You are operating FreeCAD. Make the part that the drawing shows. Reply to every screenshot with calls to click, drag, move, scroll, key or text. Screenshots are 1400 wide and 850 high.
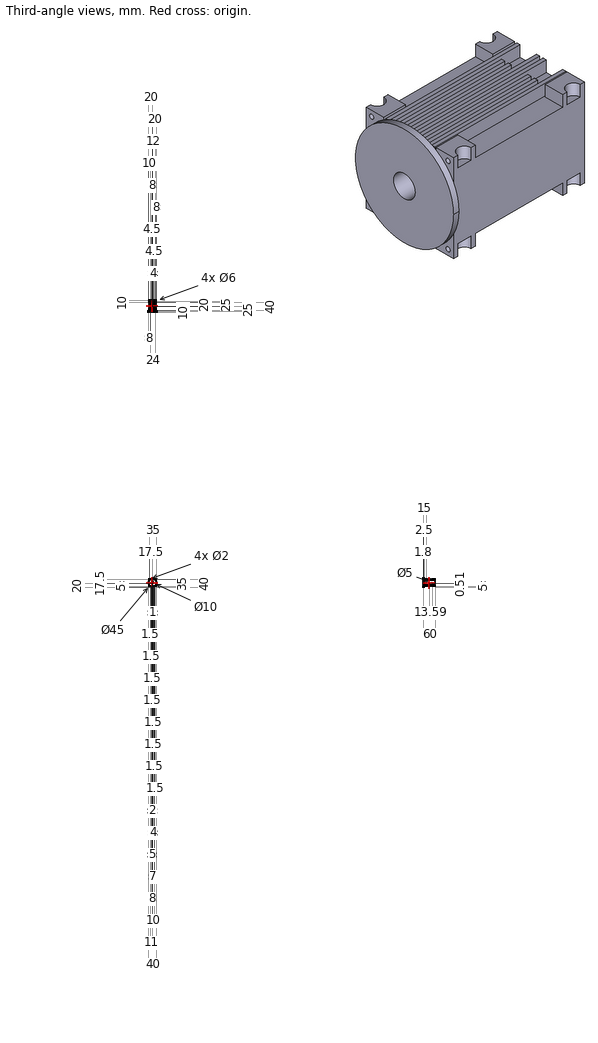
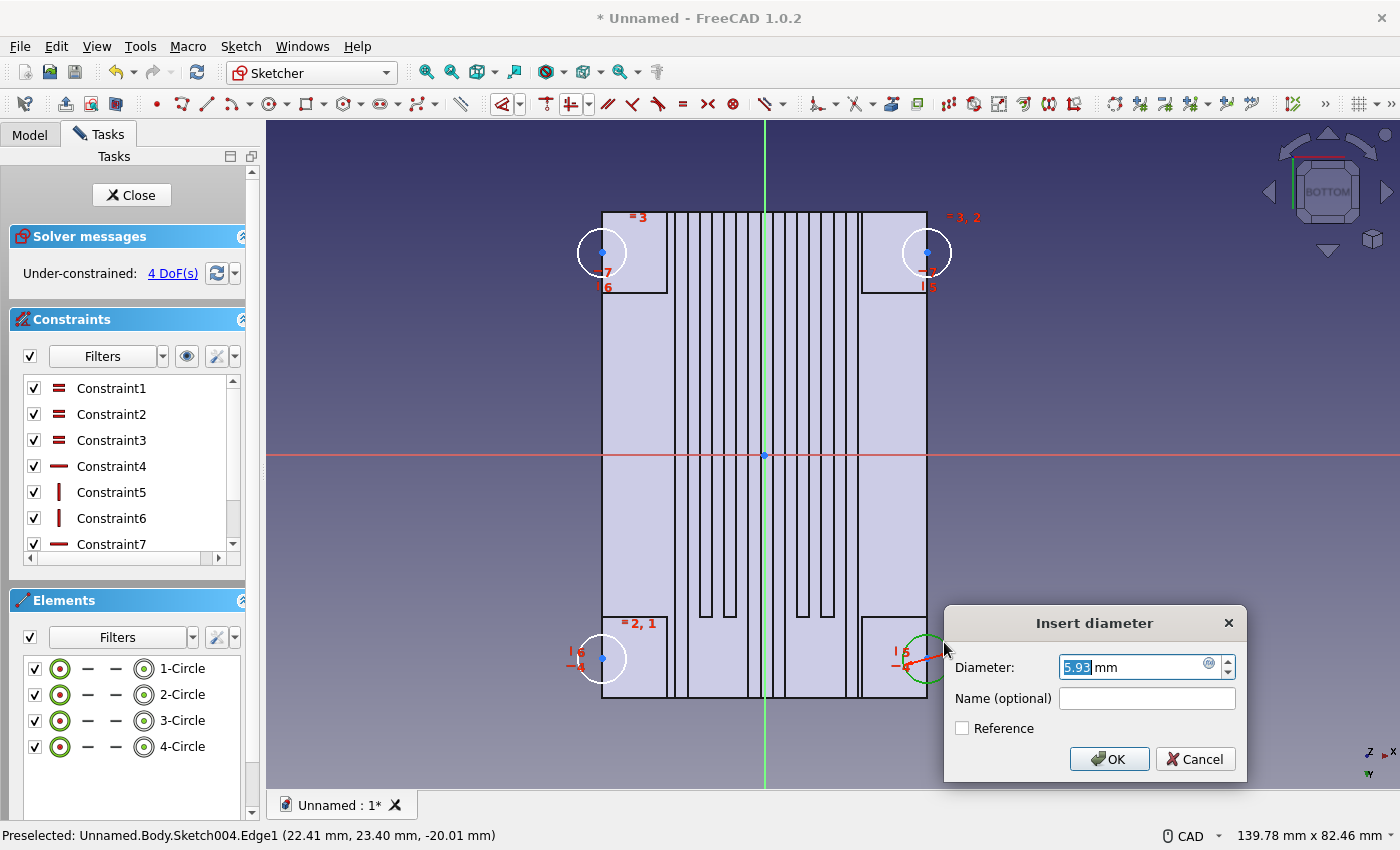
text(6)
key(Return)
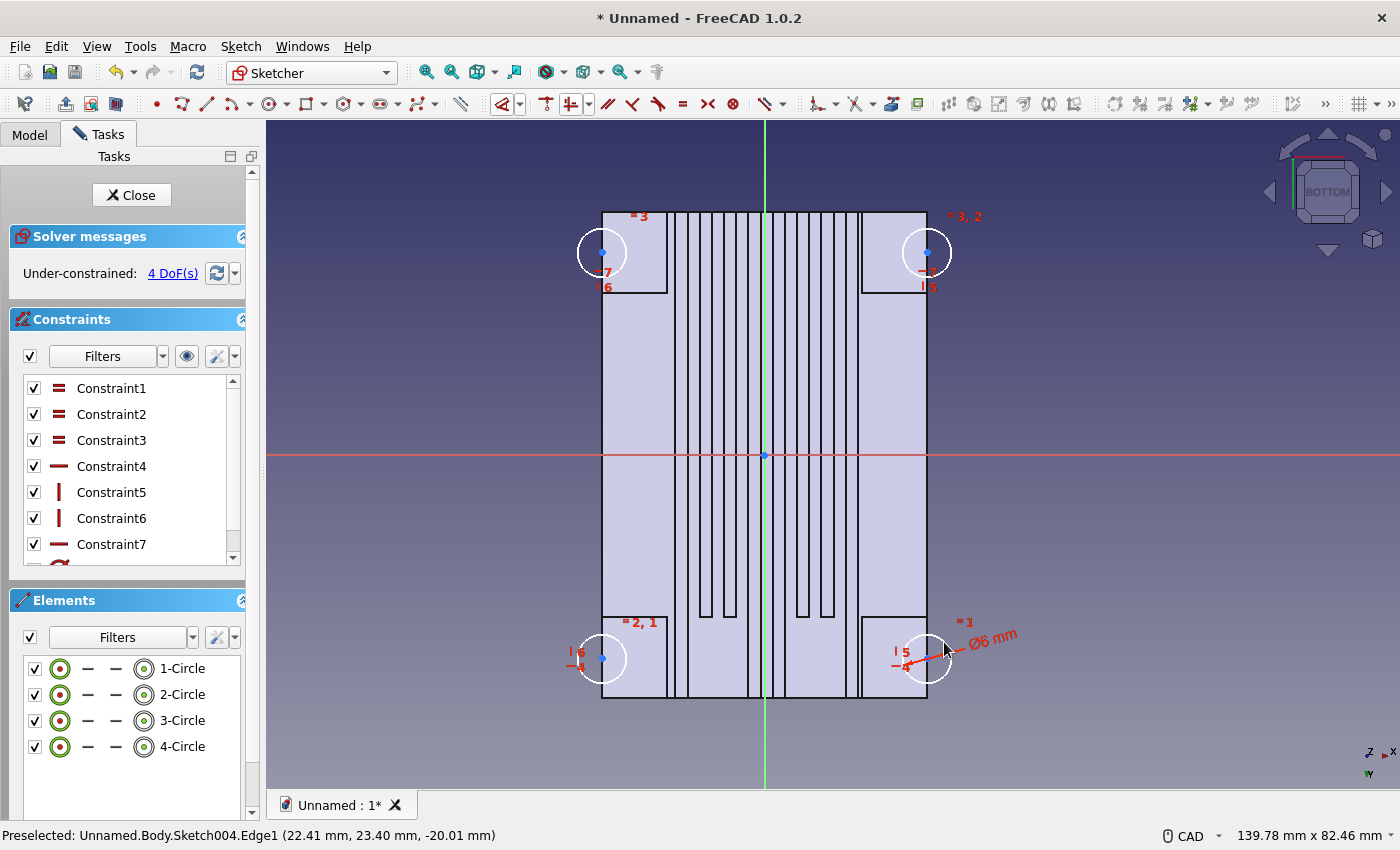
click(927, 659)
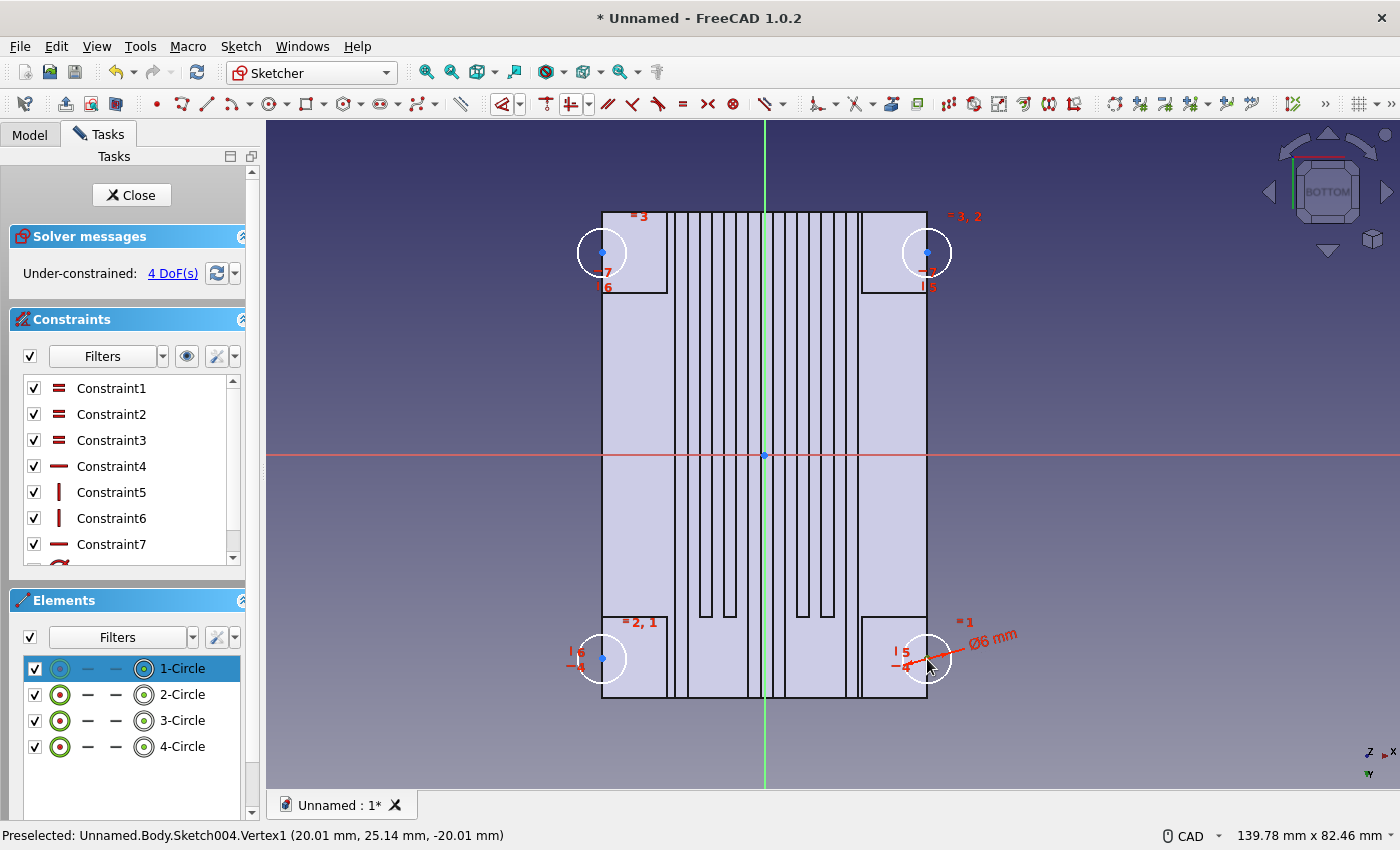
key(l)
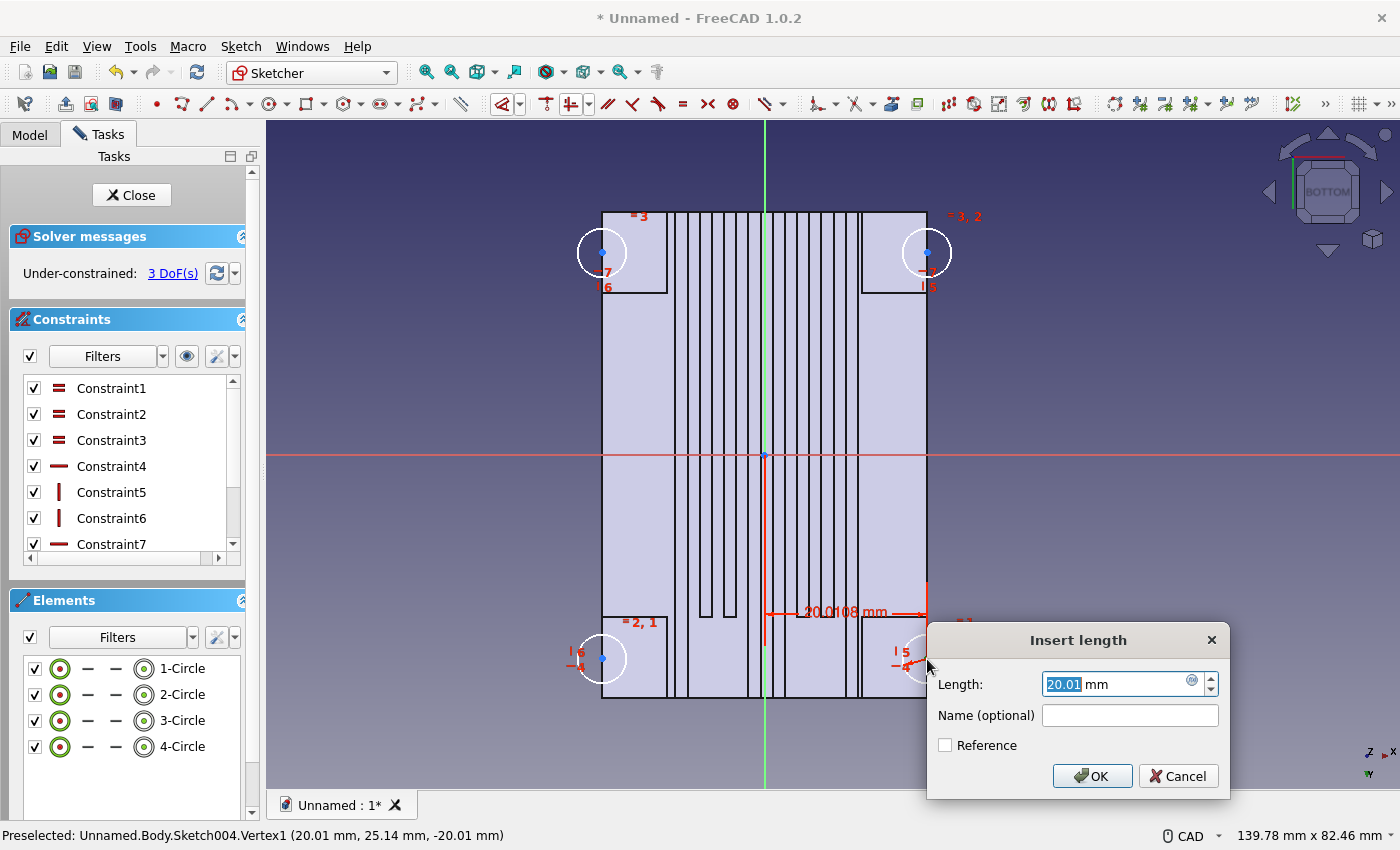
text(20)
key(Return)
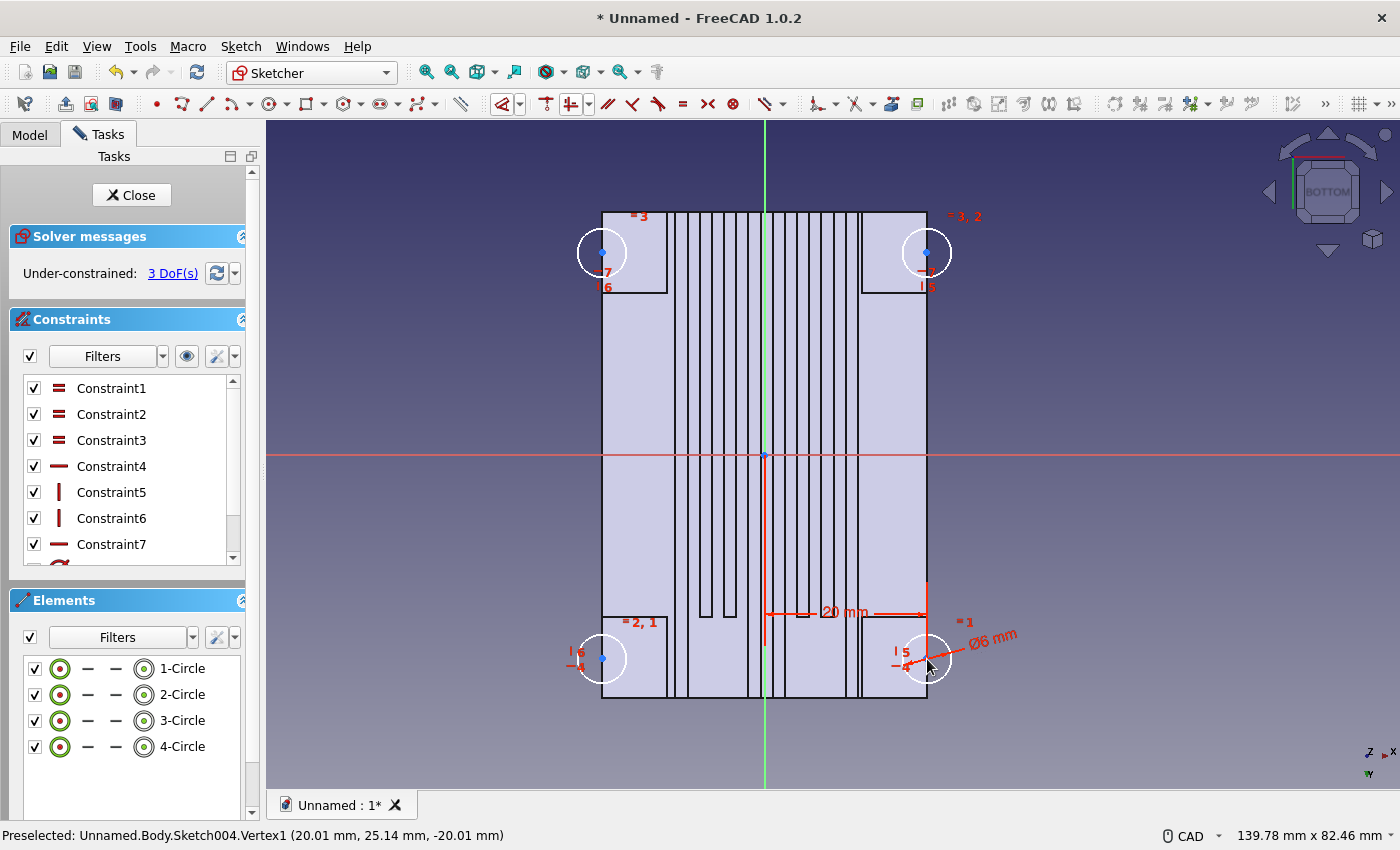
click(927, 659)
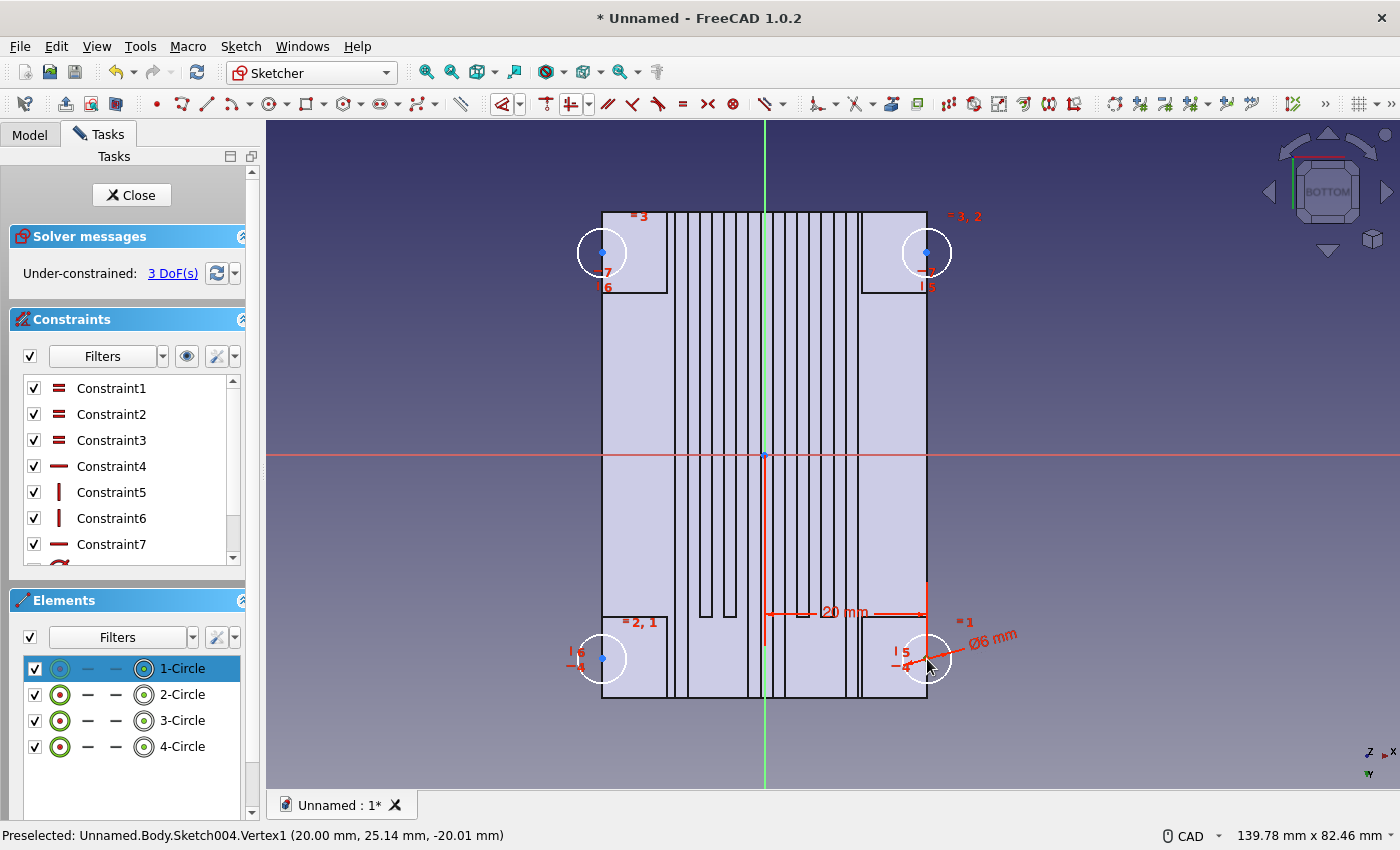
key(i)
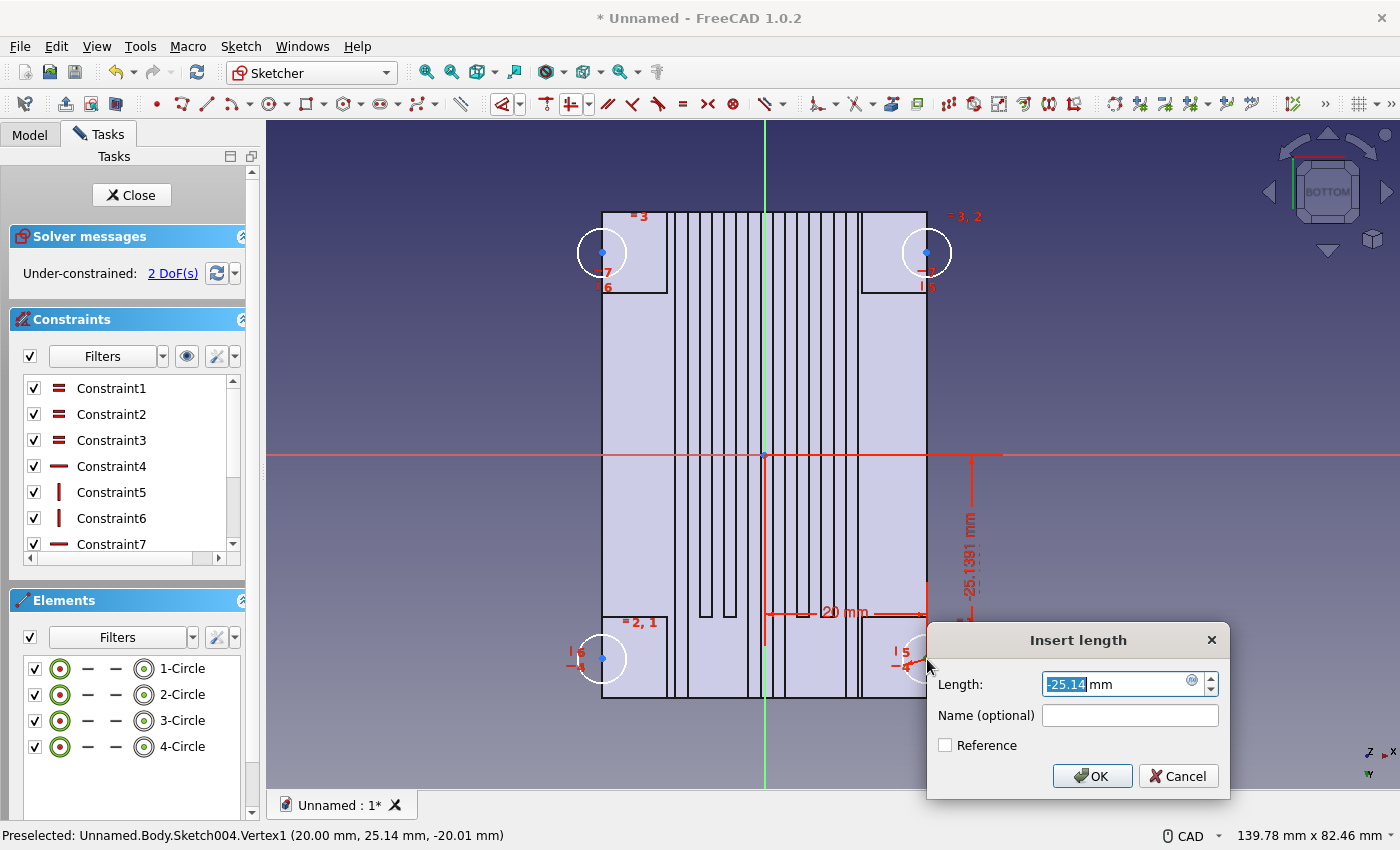
text(-25)
key(Return)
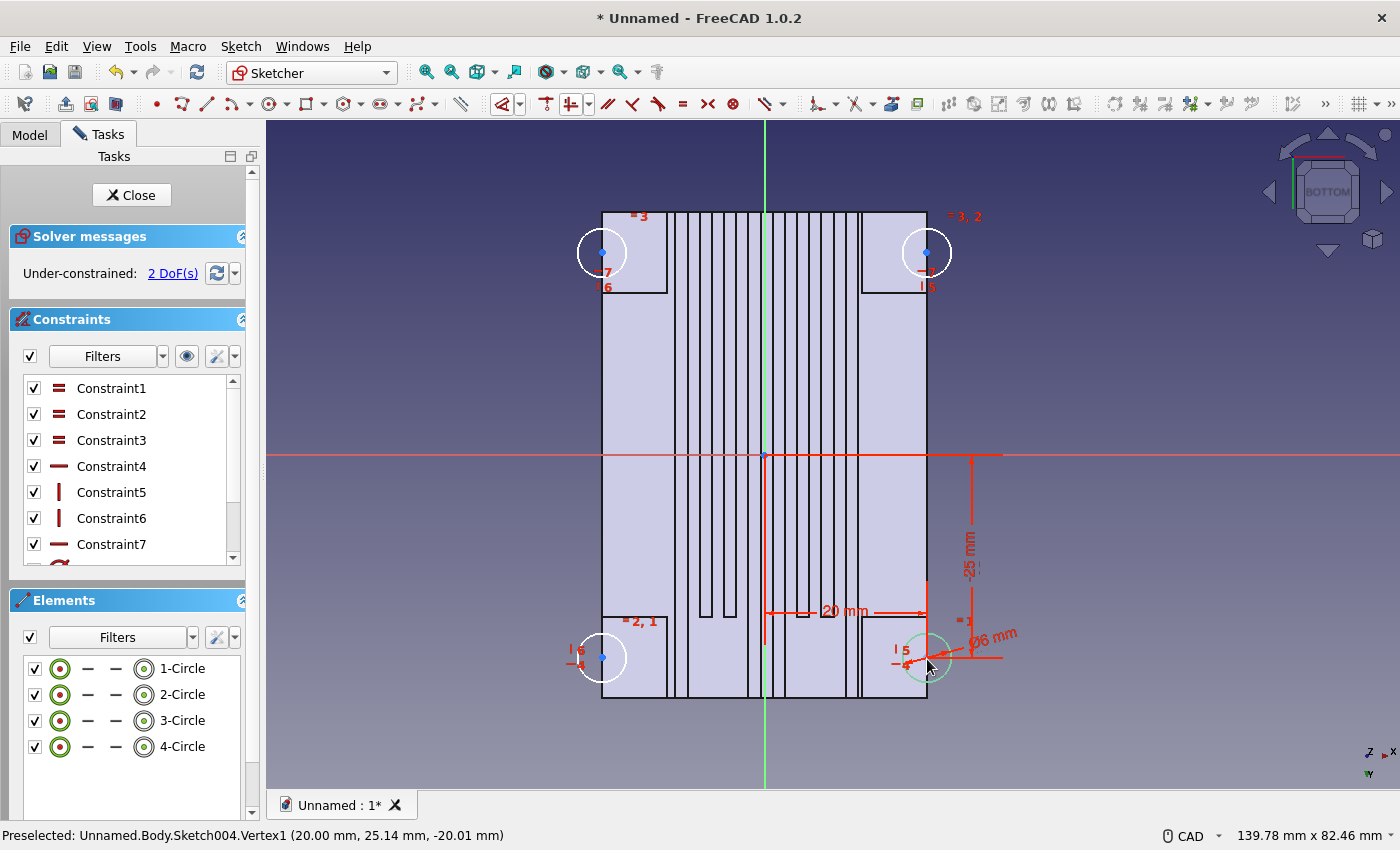
click(602, 658)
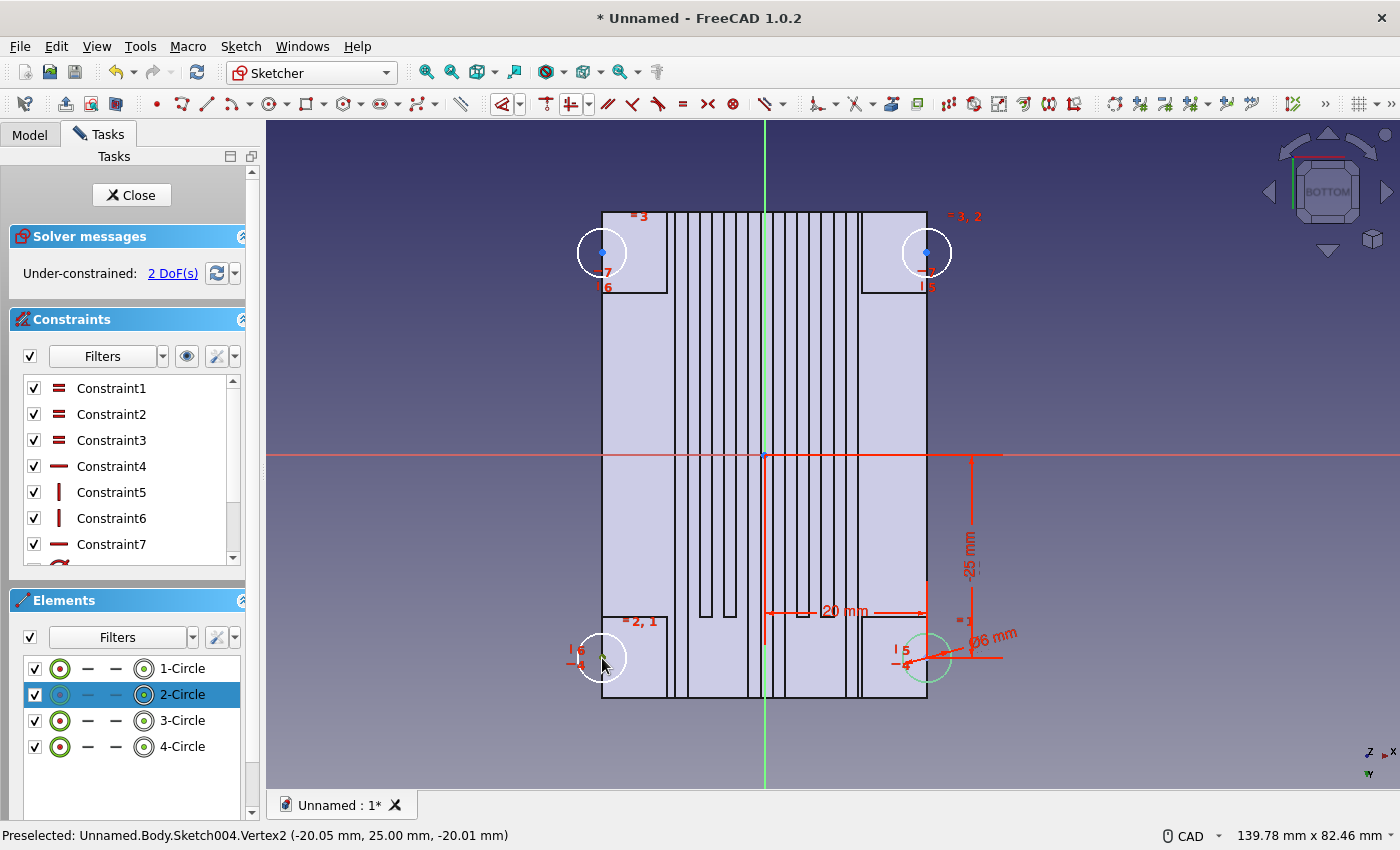
key(l)